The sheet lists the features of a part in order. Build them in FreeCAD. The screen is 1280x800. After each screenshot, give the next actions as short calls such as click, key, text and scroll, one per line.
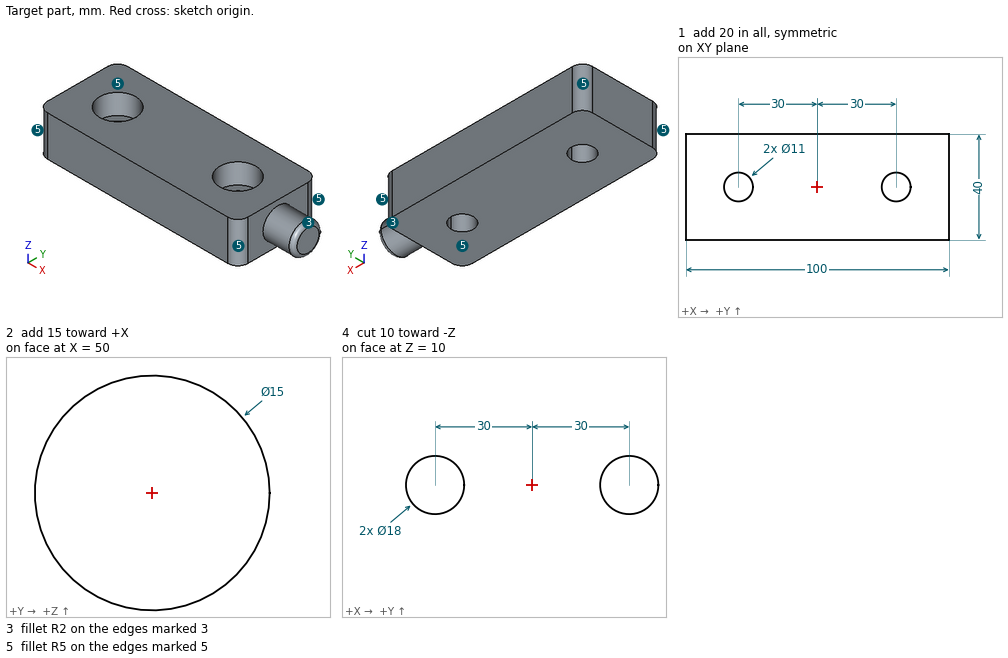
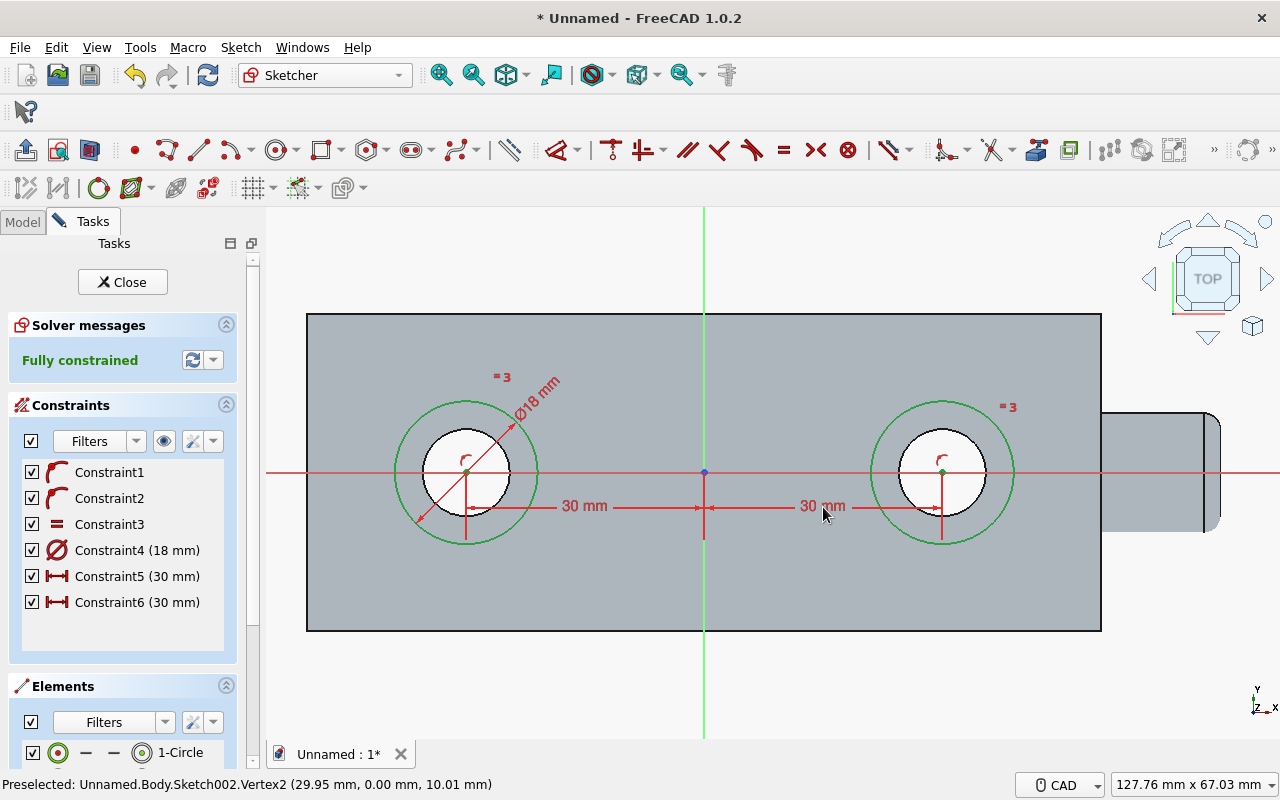
click(123, 282)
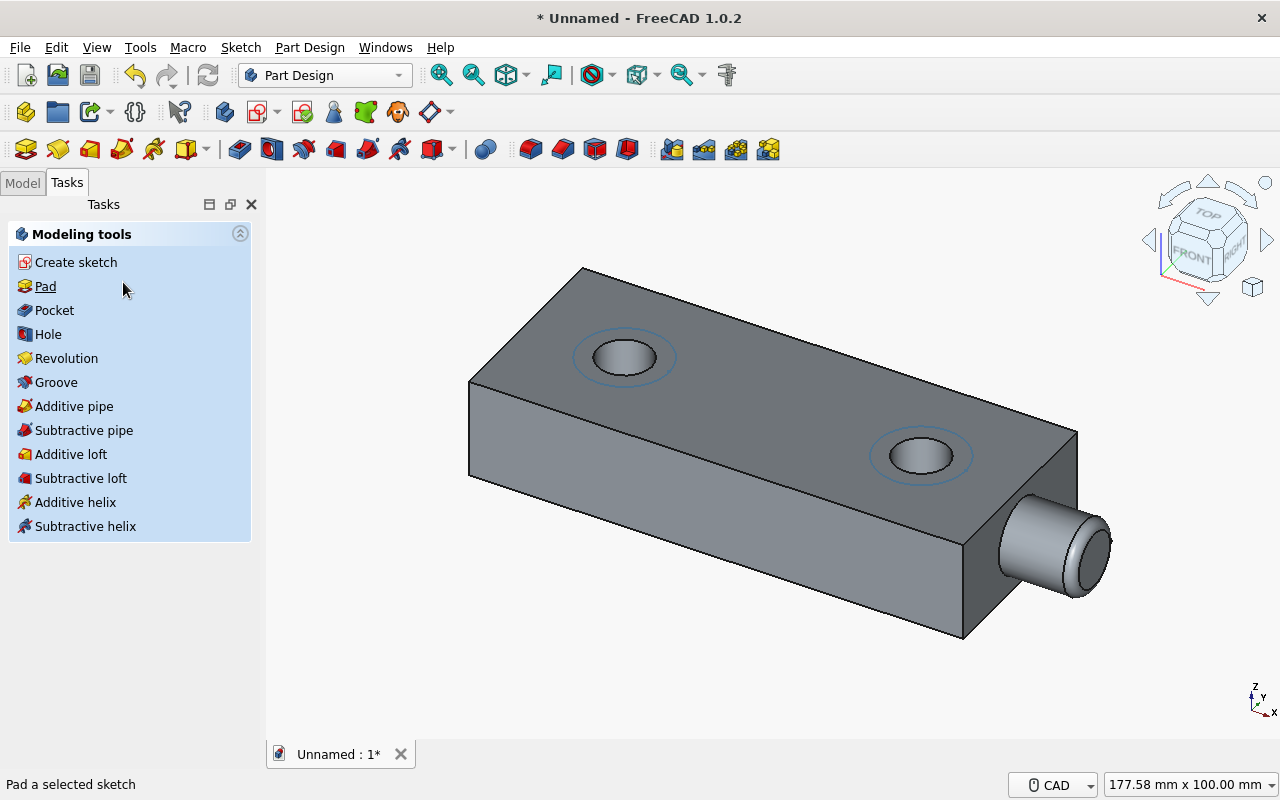
click(240, 150)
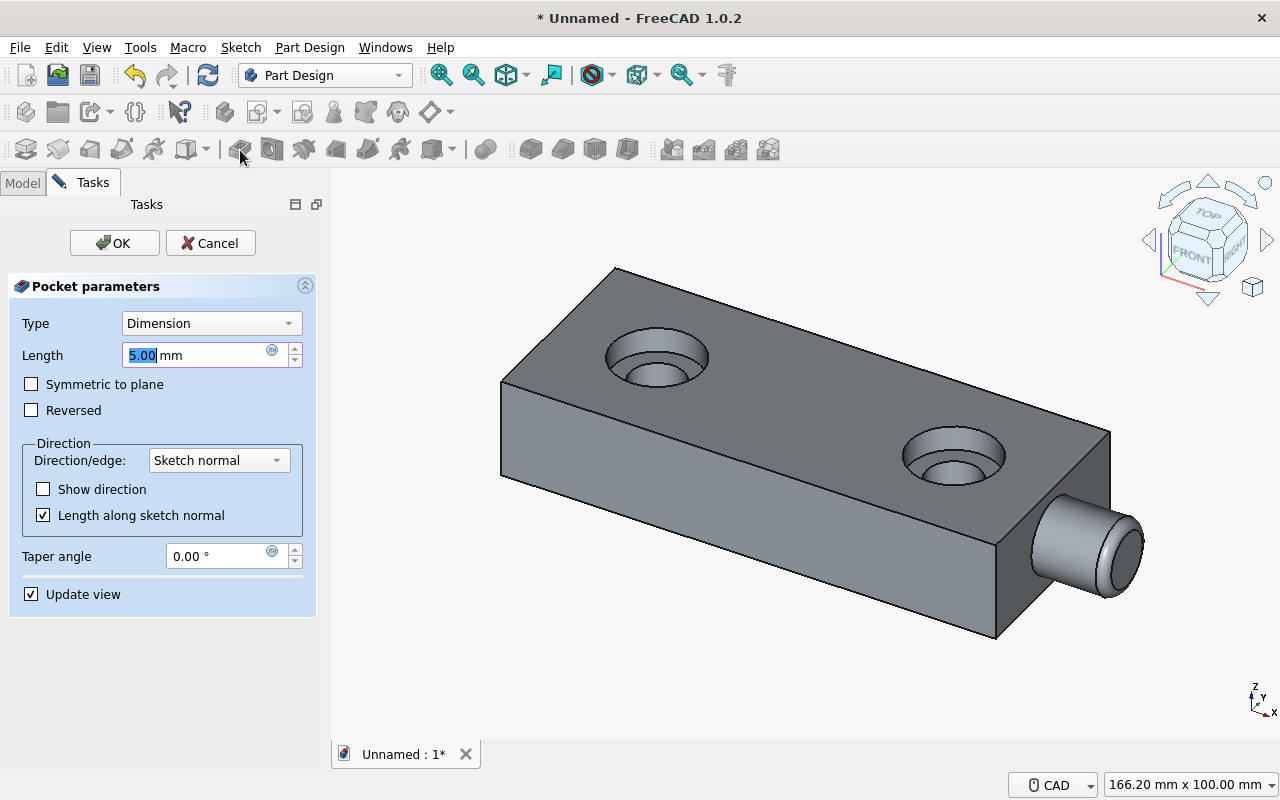
text(10)
key(Tab)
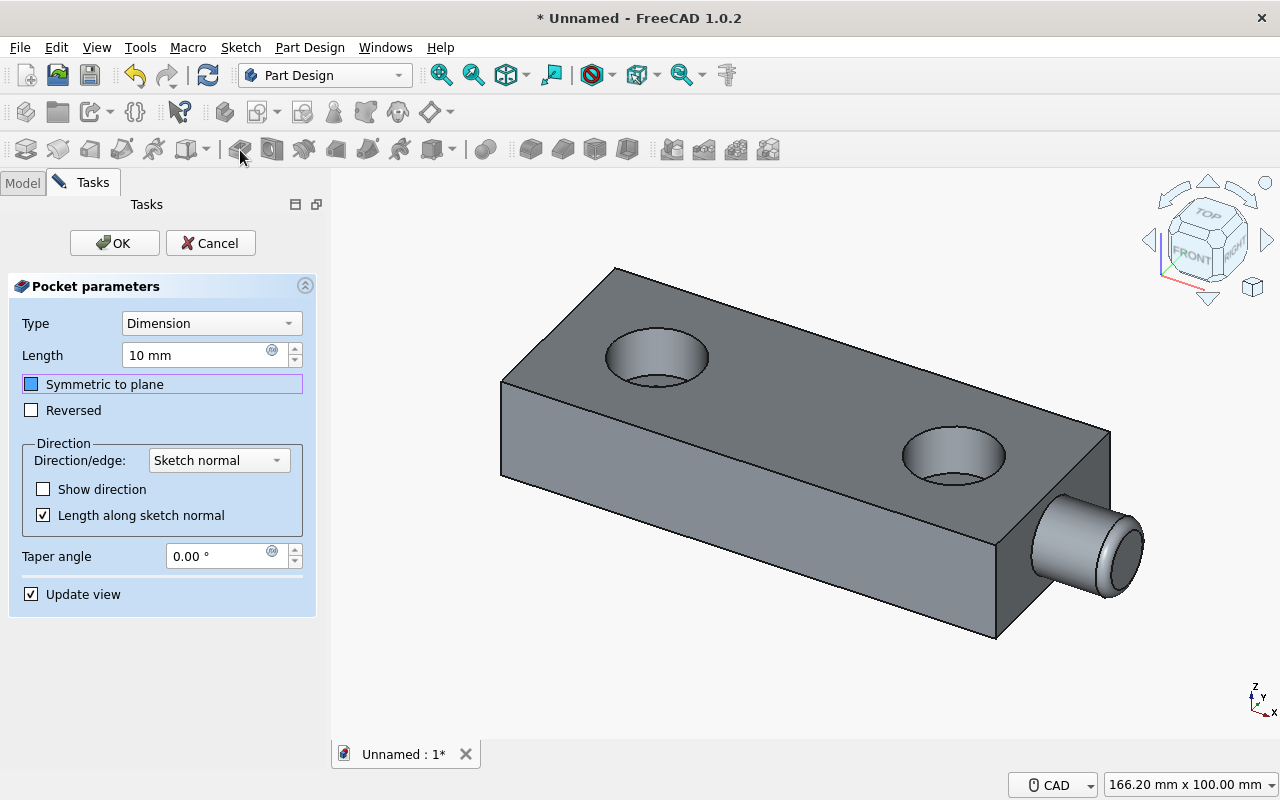
click(115, 243)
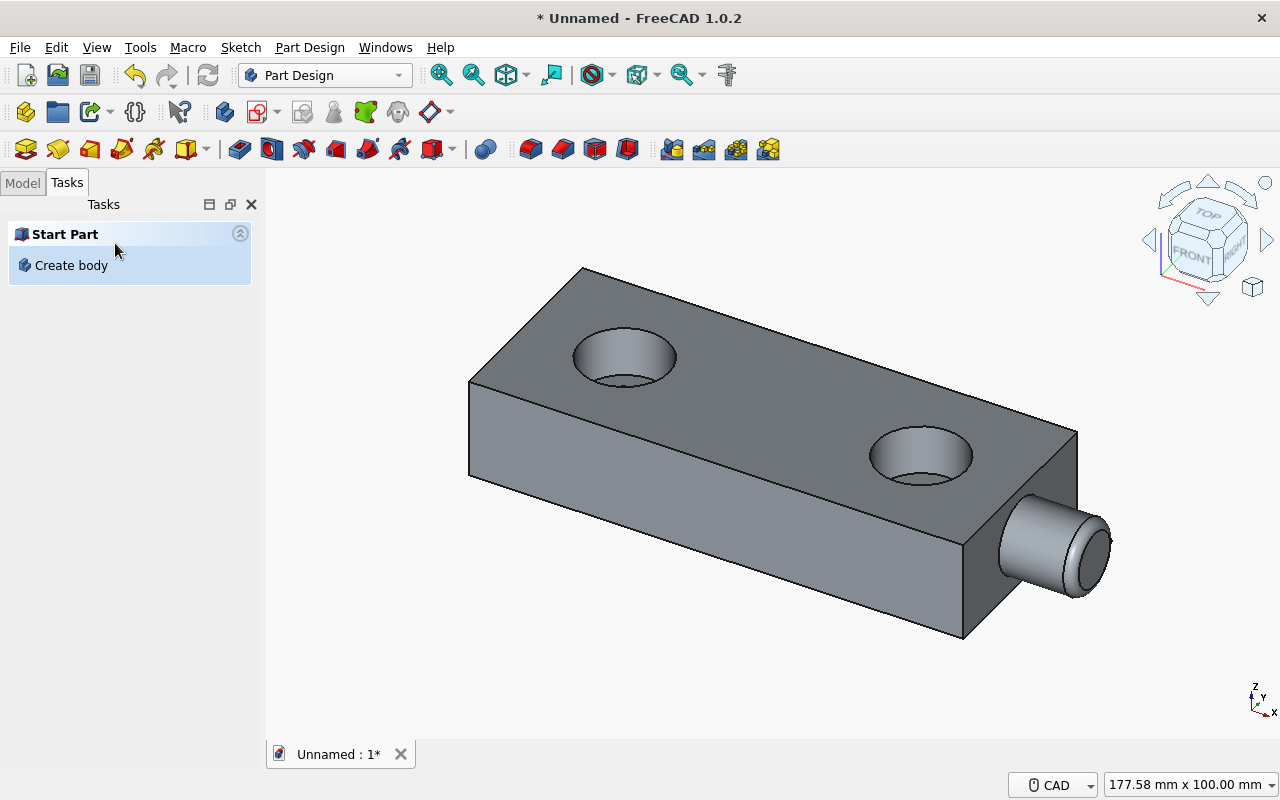
click(963, 591)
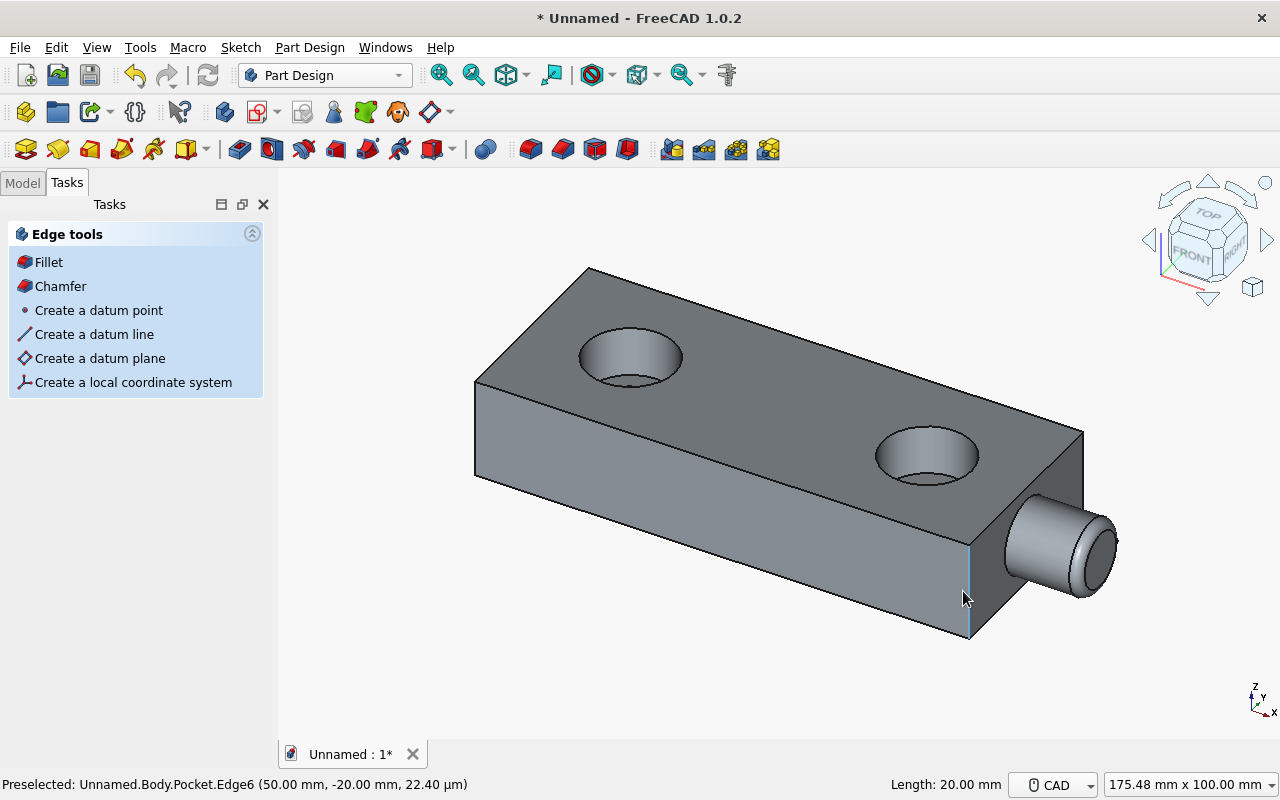
key(0)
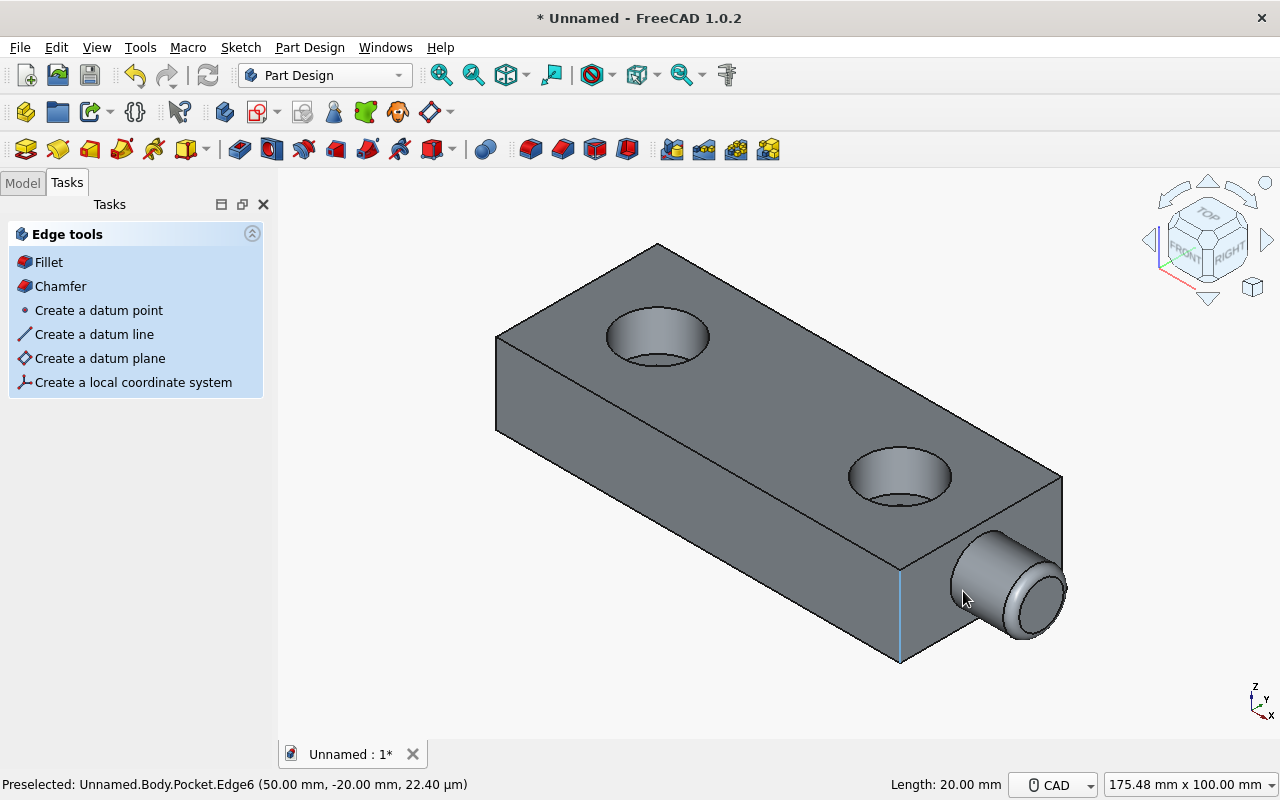
key(2)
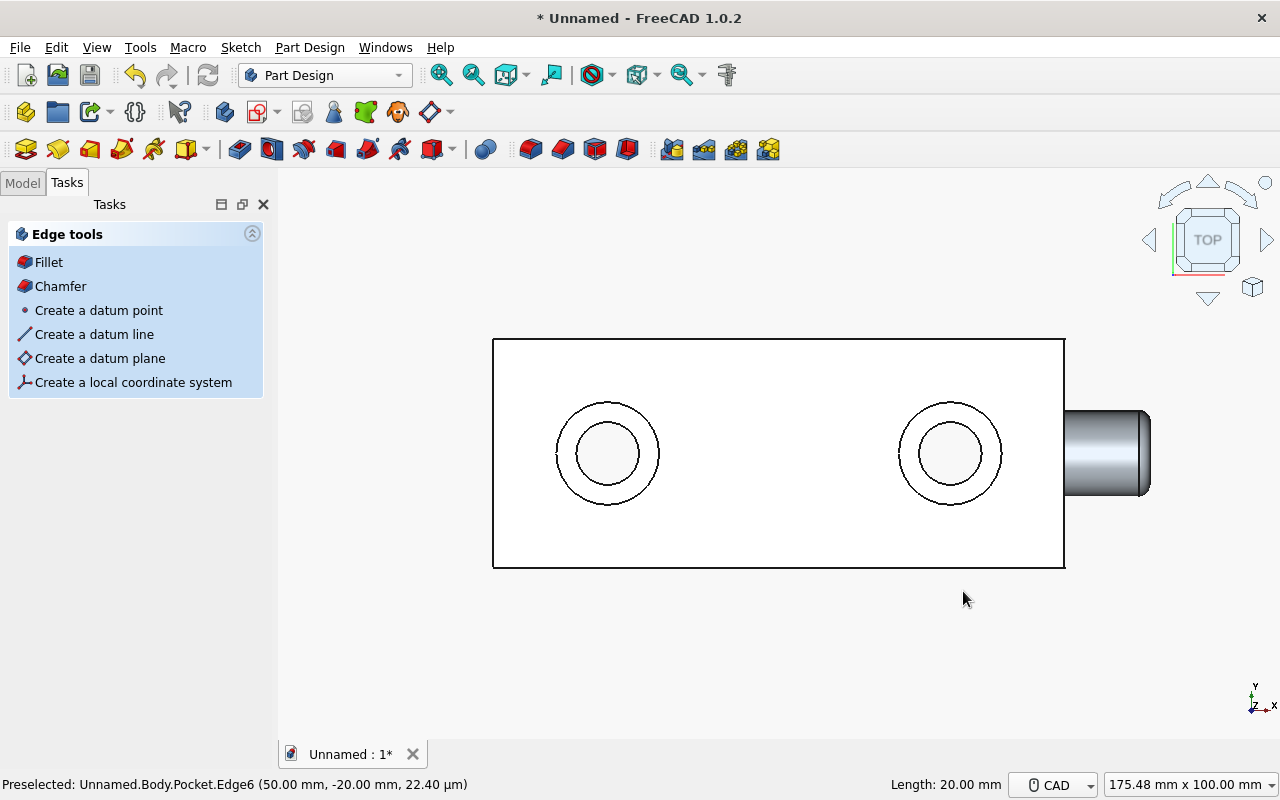
key(1)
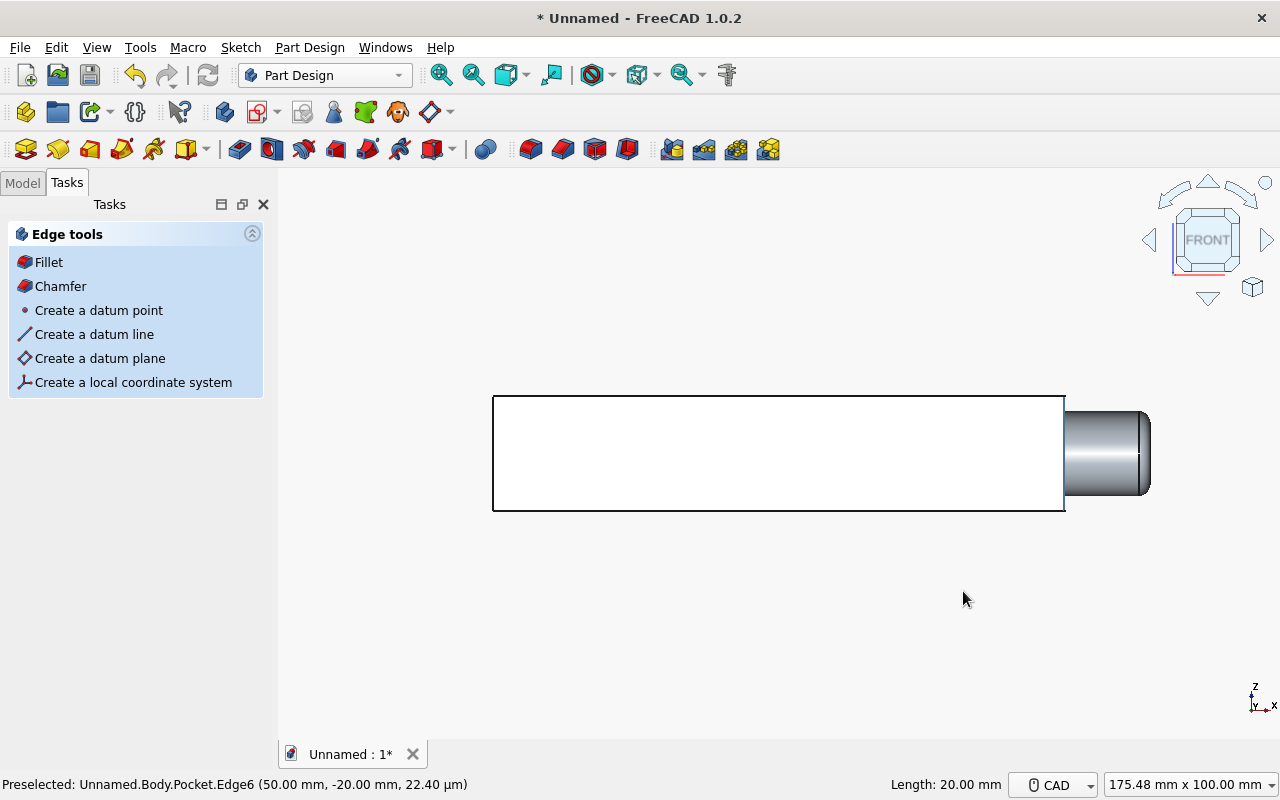
click(493, 452, ctrl)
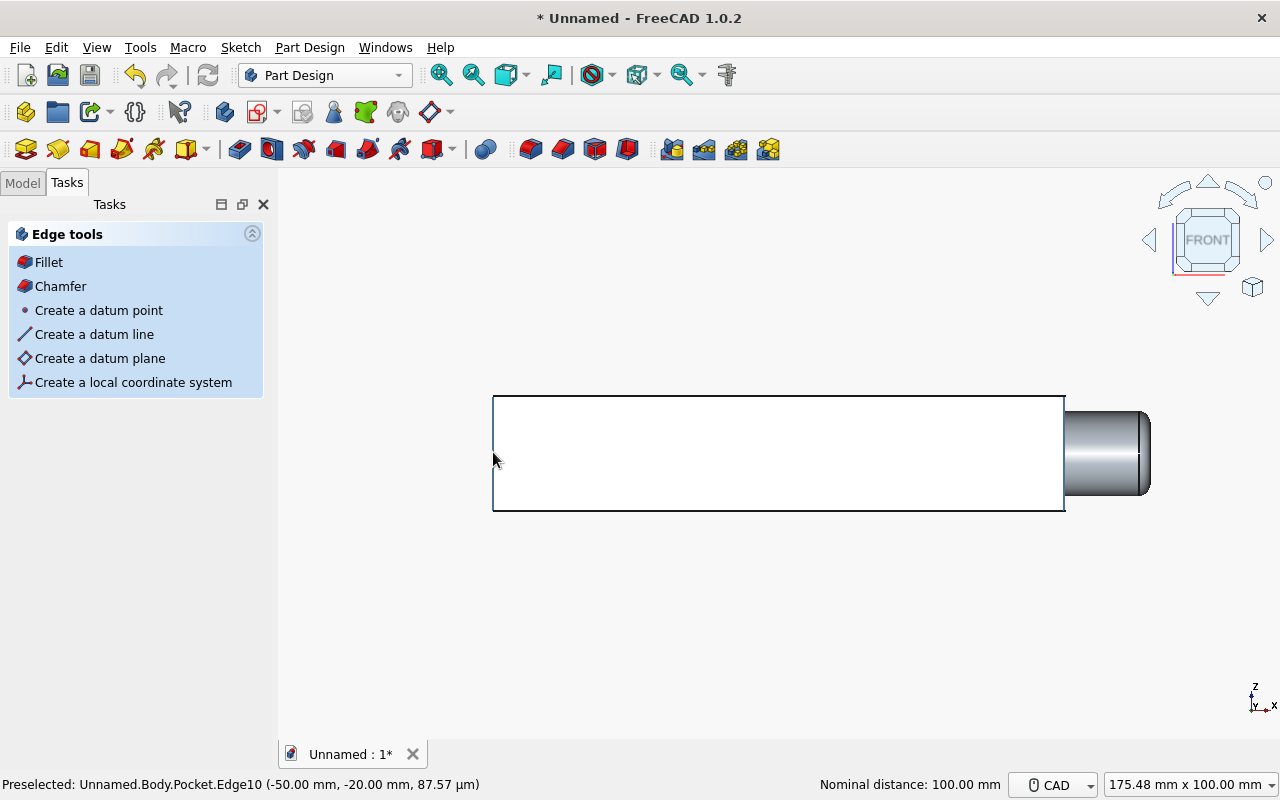
key(3)